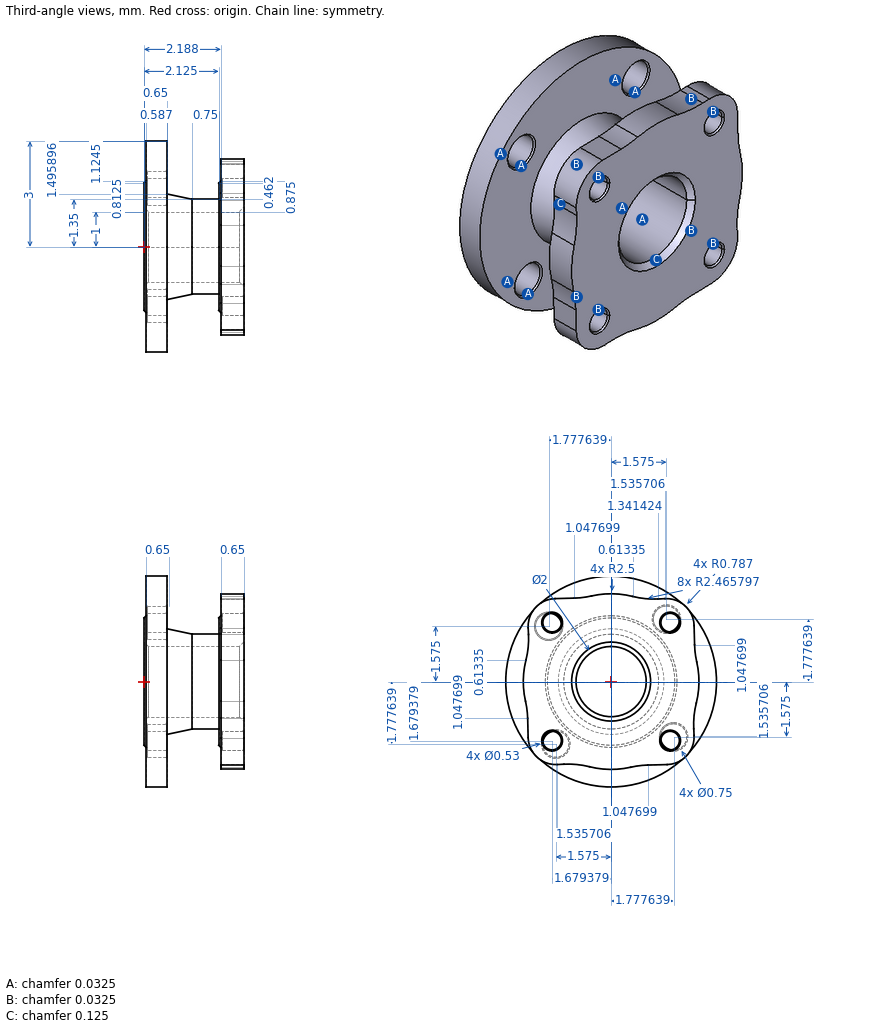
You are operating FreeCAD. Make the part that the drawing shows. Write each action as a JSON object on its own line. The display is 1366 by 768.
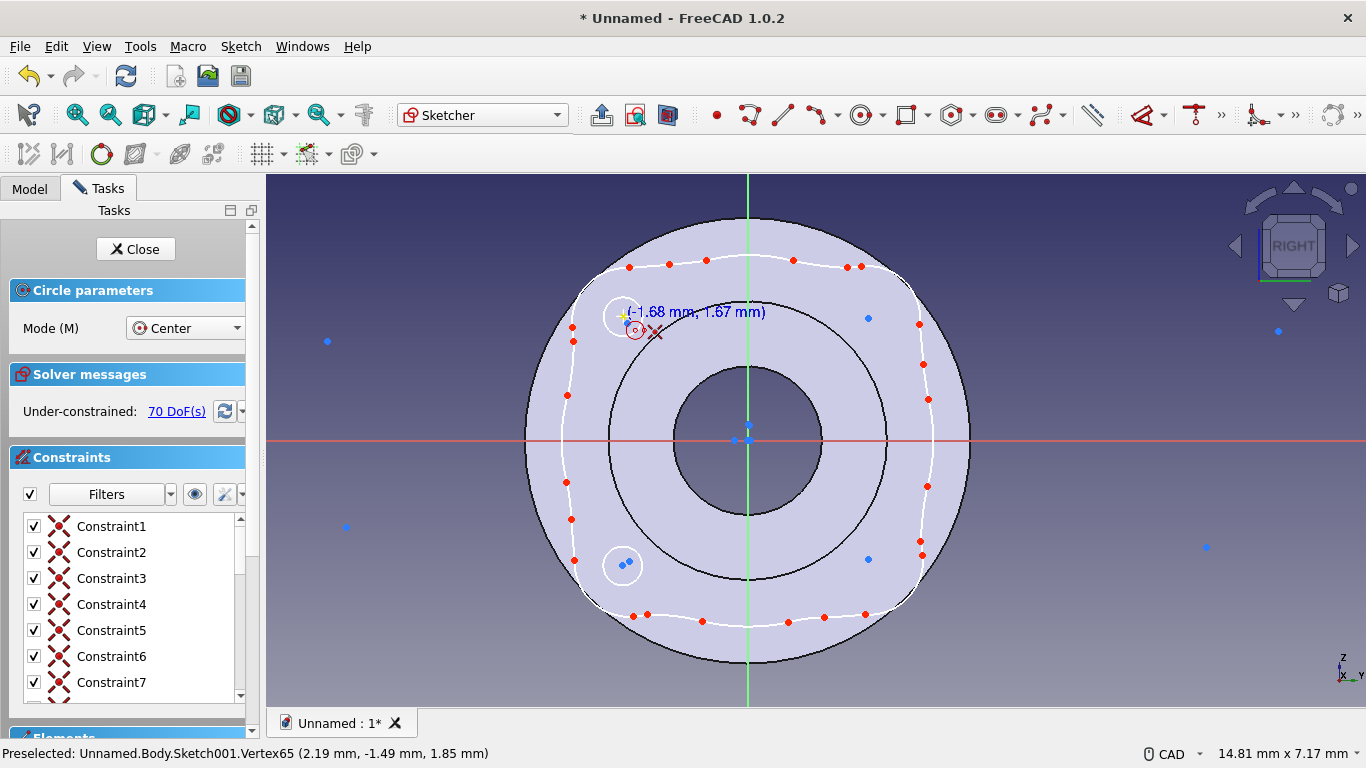
{"action": "scroll", "coordinate": [872, 565], "scroll_direction": "up", "scroll_amount": 2}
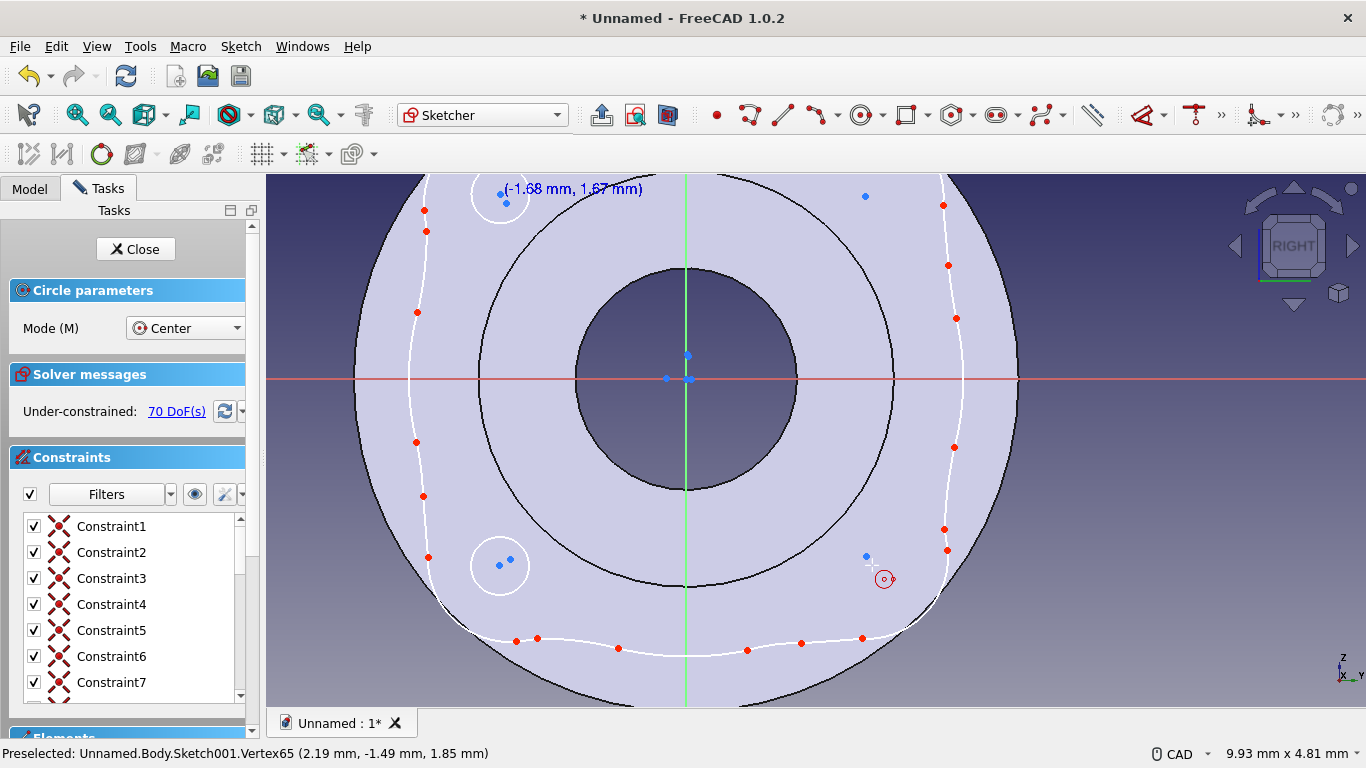
{"action": "left_click", "coordinate": [872, 565]}
{"action": "left_click", "coordinate": [893, 545]}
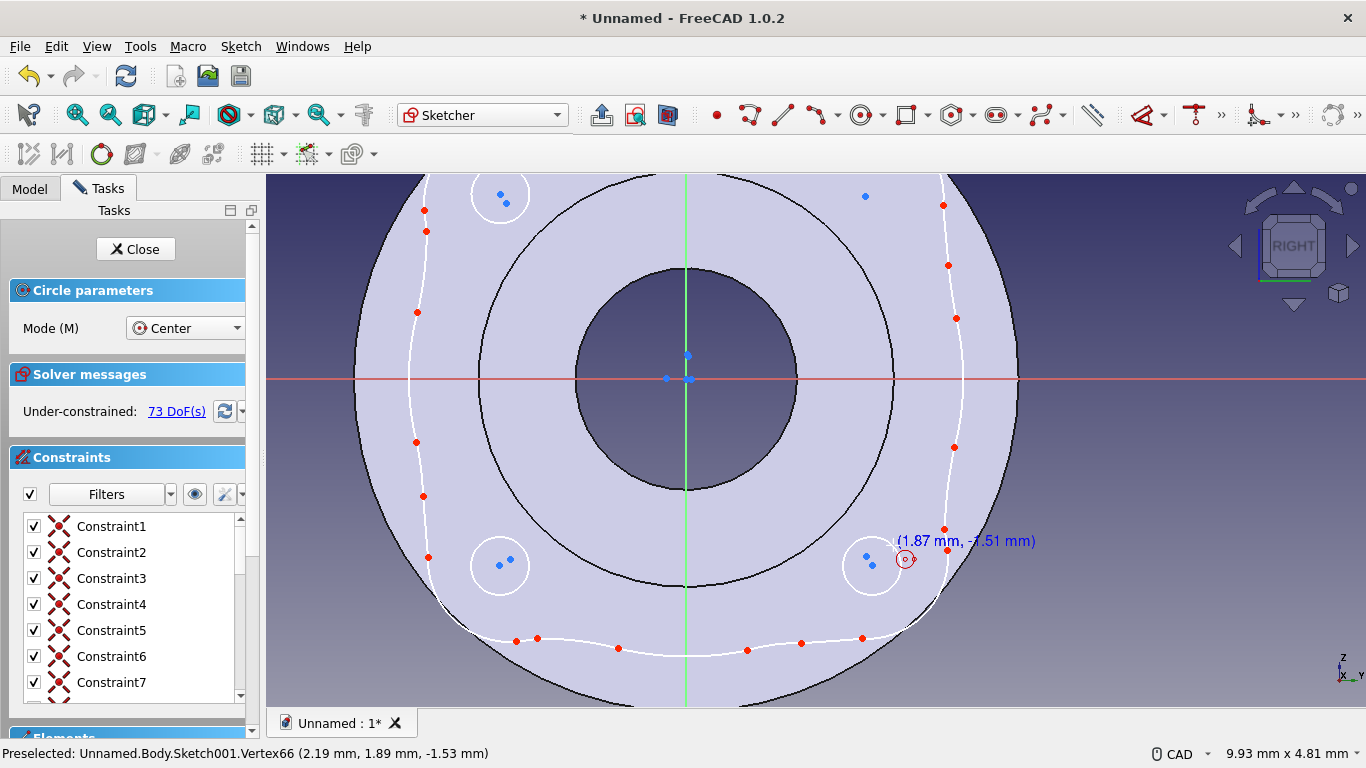
{"action": "left_click", "coordinate": [686, 379]}
{"action": "left_click", "coordinate": [765, 301]}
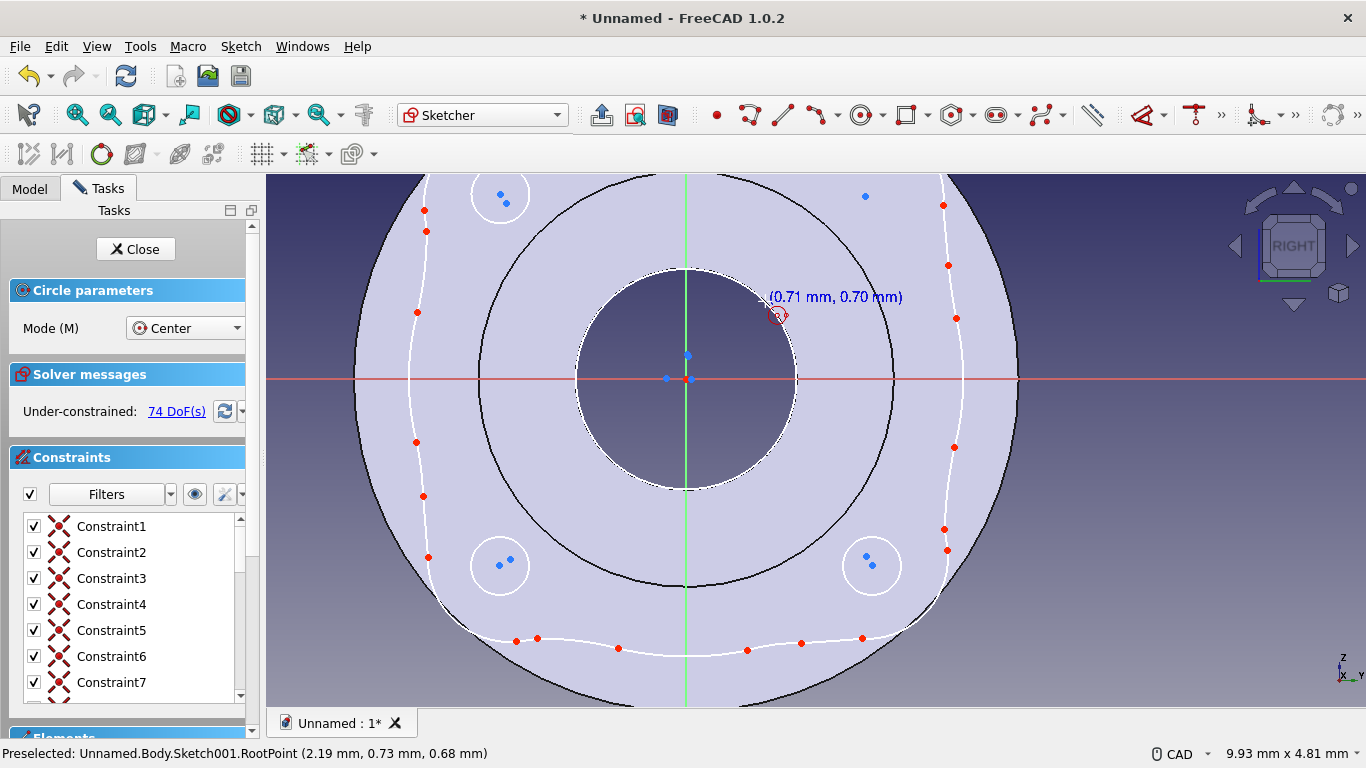
{"action": "scroll", "coordinate": [872, 565], "scroll_direction": "down", "scroll_amount": 2}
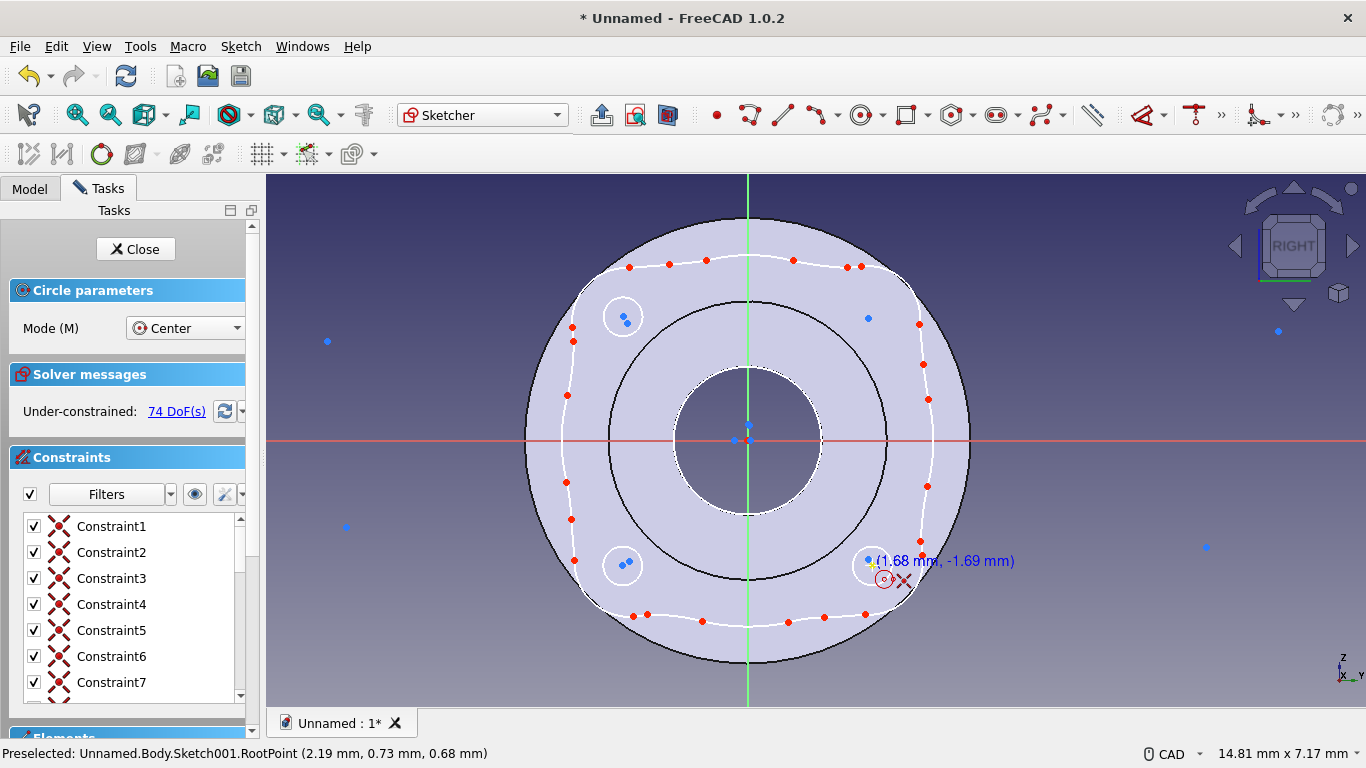
{"action": "scroll", "coordinate": [872, 316], "scroll_direction": "up", "scroll_amount": 2}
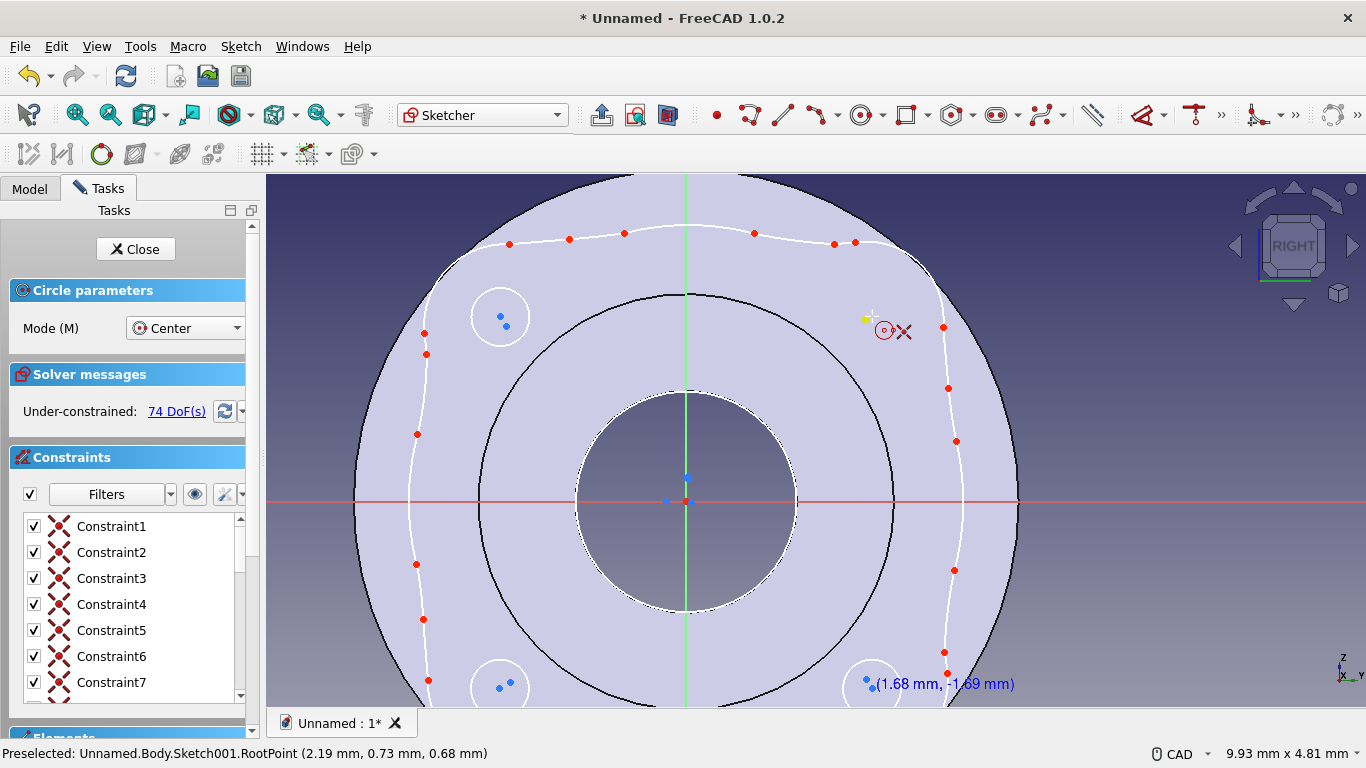
{"action": "left_click", "coordinate": [872, 316]}
{"action": "left_click", "coordinate": [893, 295]}
{"action": "key", "text": "Escape"}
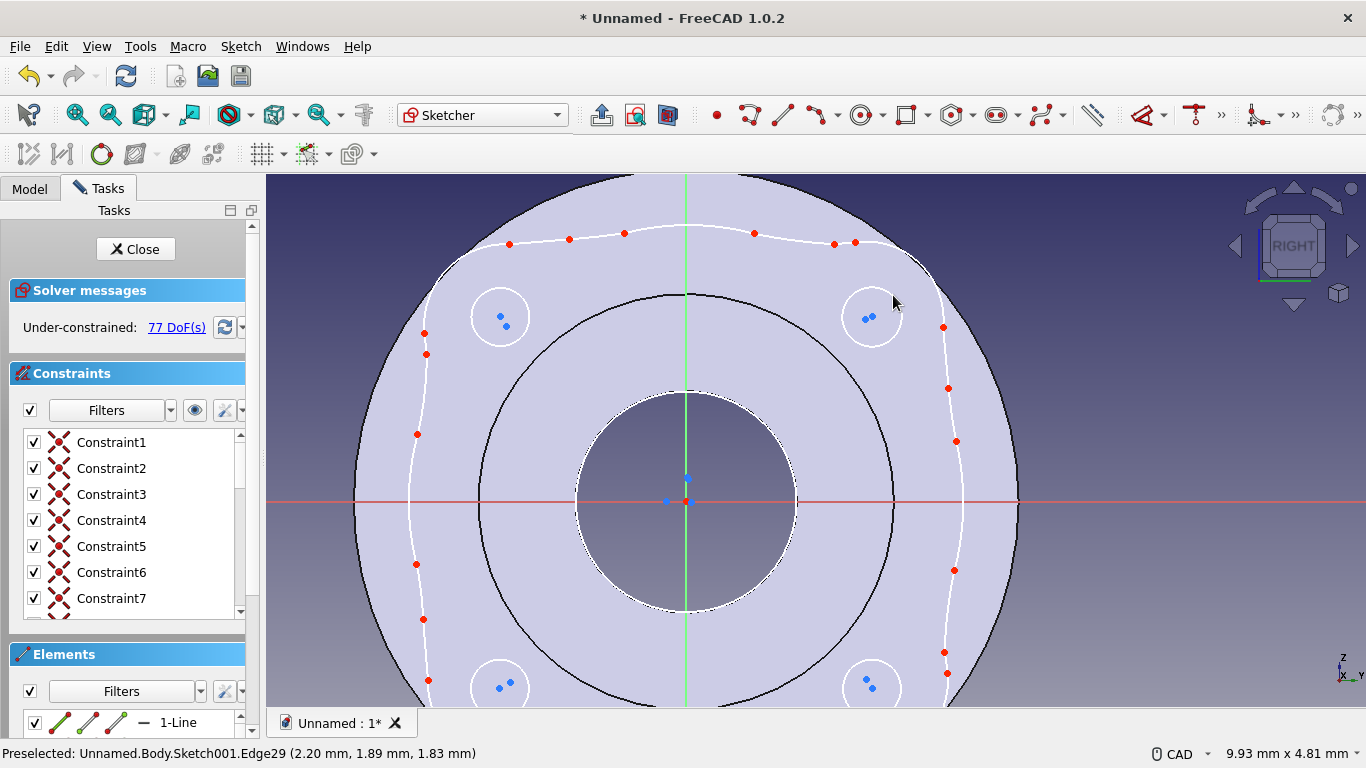
{"action": "left_click", "coordinate": [947, 370]}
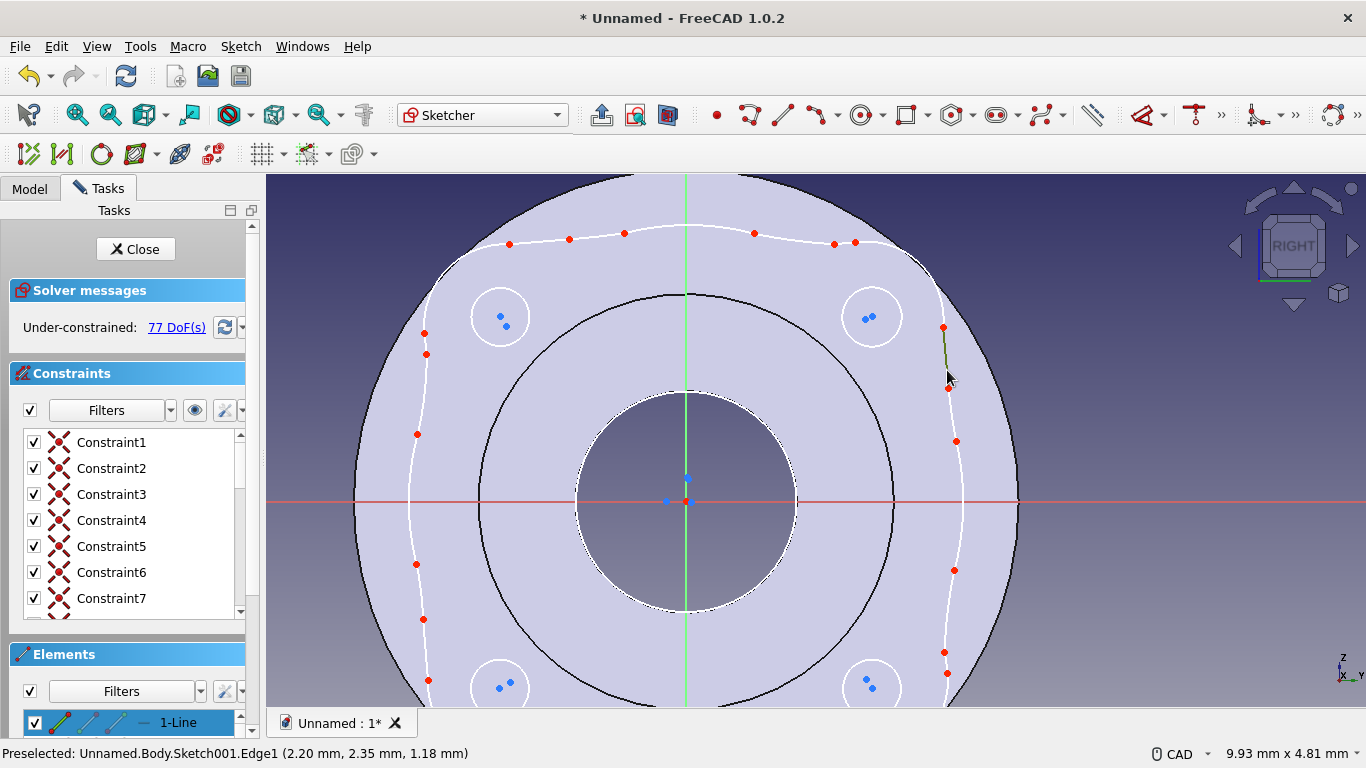
{"action": "left_click", "coordinate": [936, 287]}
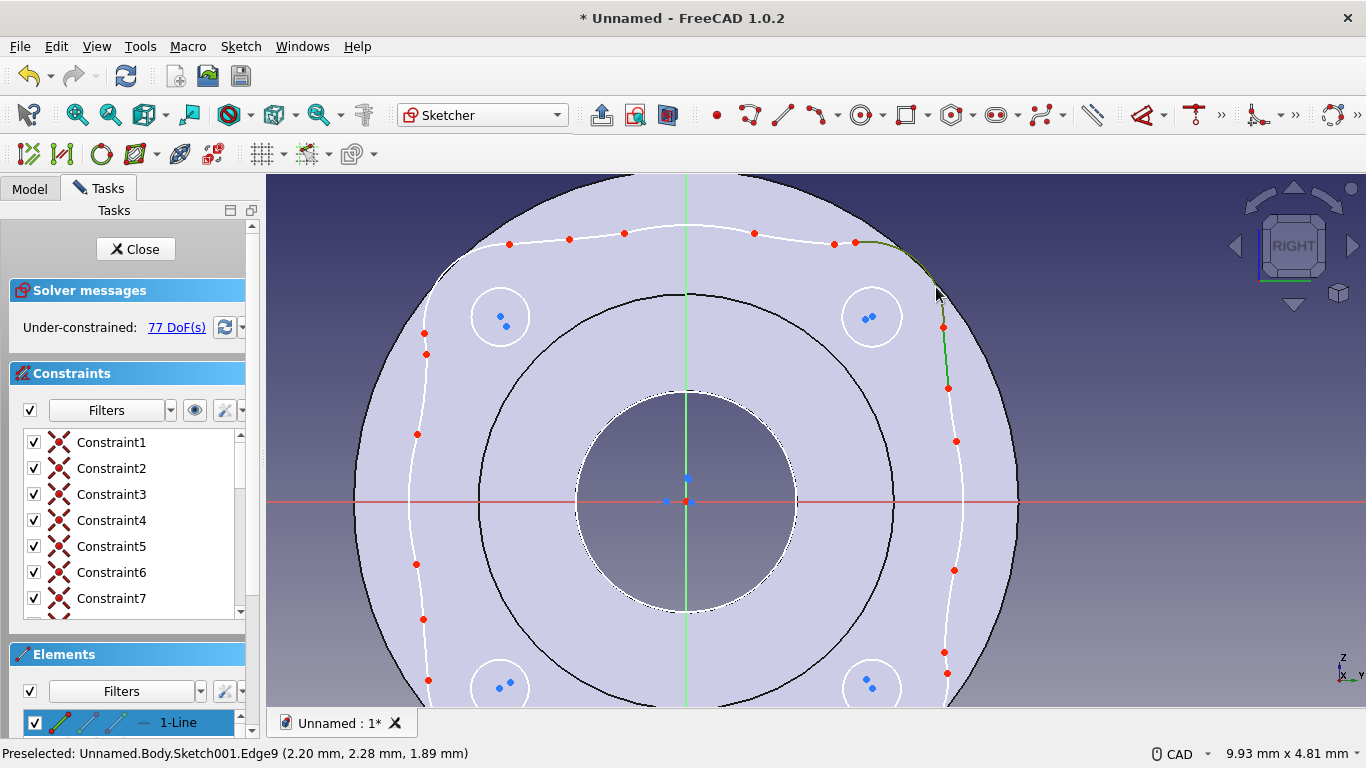
{"action": "key", "text": "t"}